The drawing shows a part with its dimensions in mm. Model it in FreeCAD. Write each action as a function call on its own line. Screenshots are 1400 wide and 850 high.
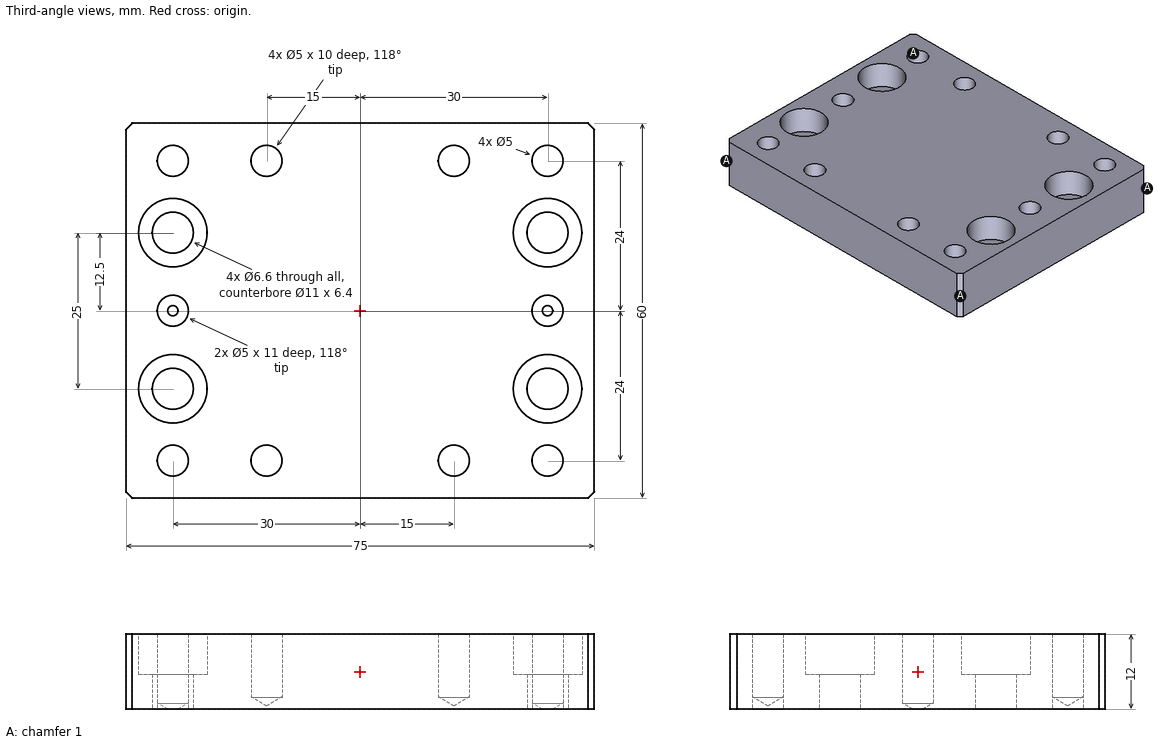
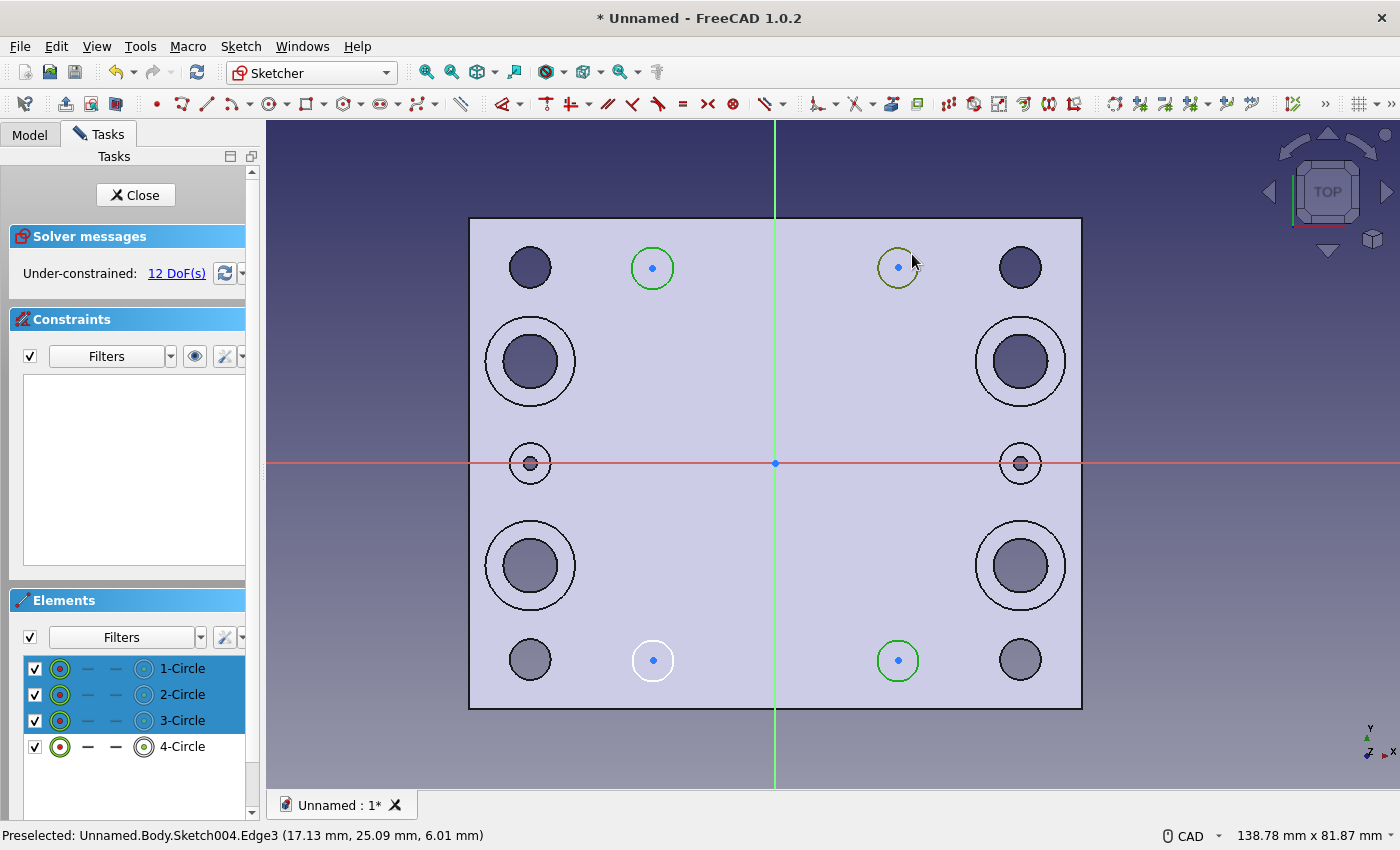
click(667, 646)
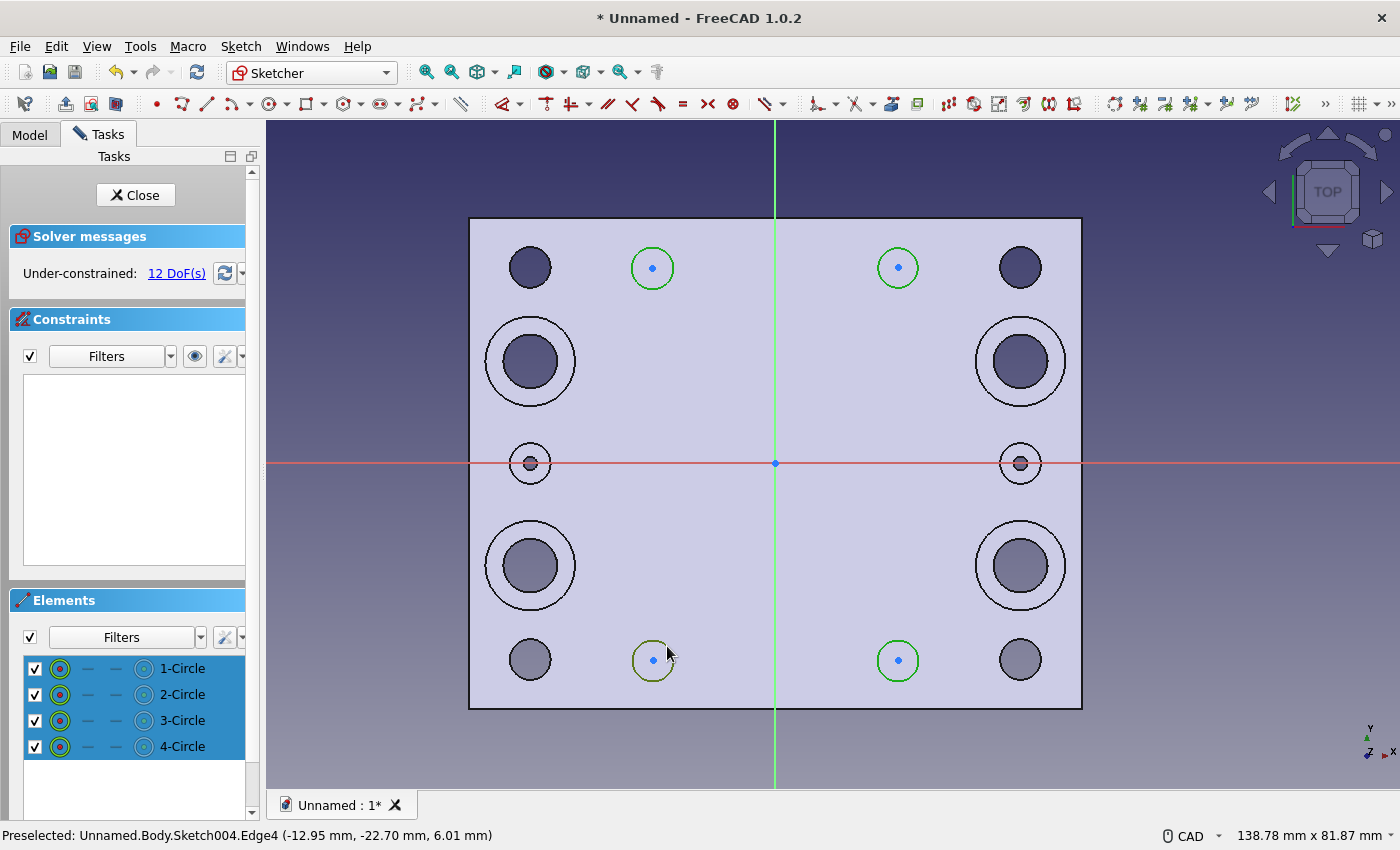
key(e)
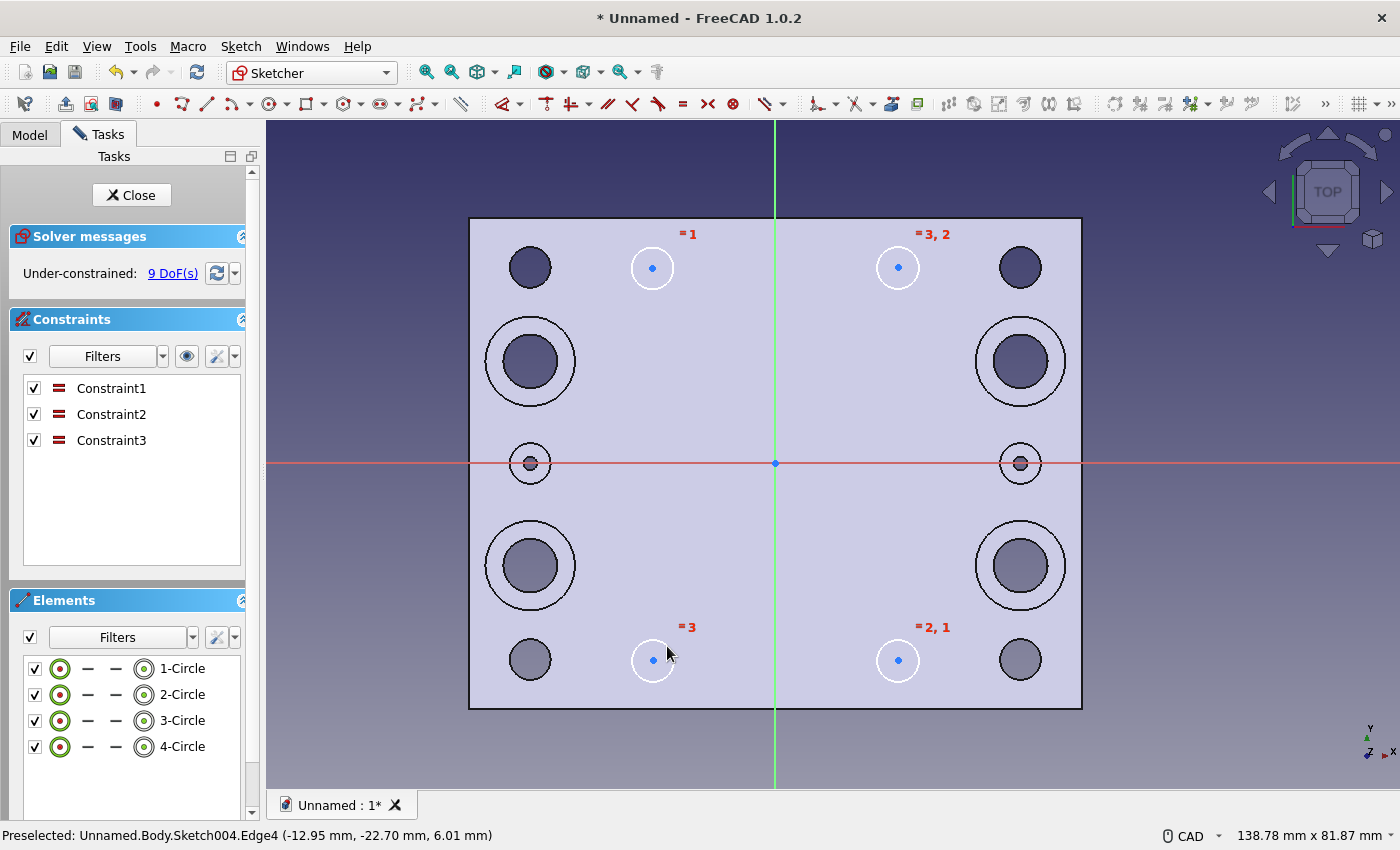
key(d)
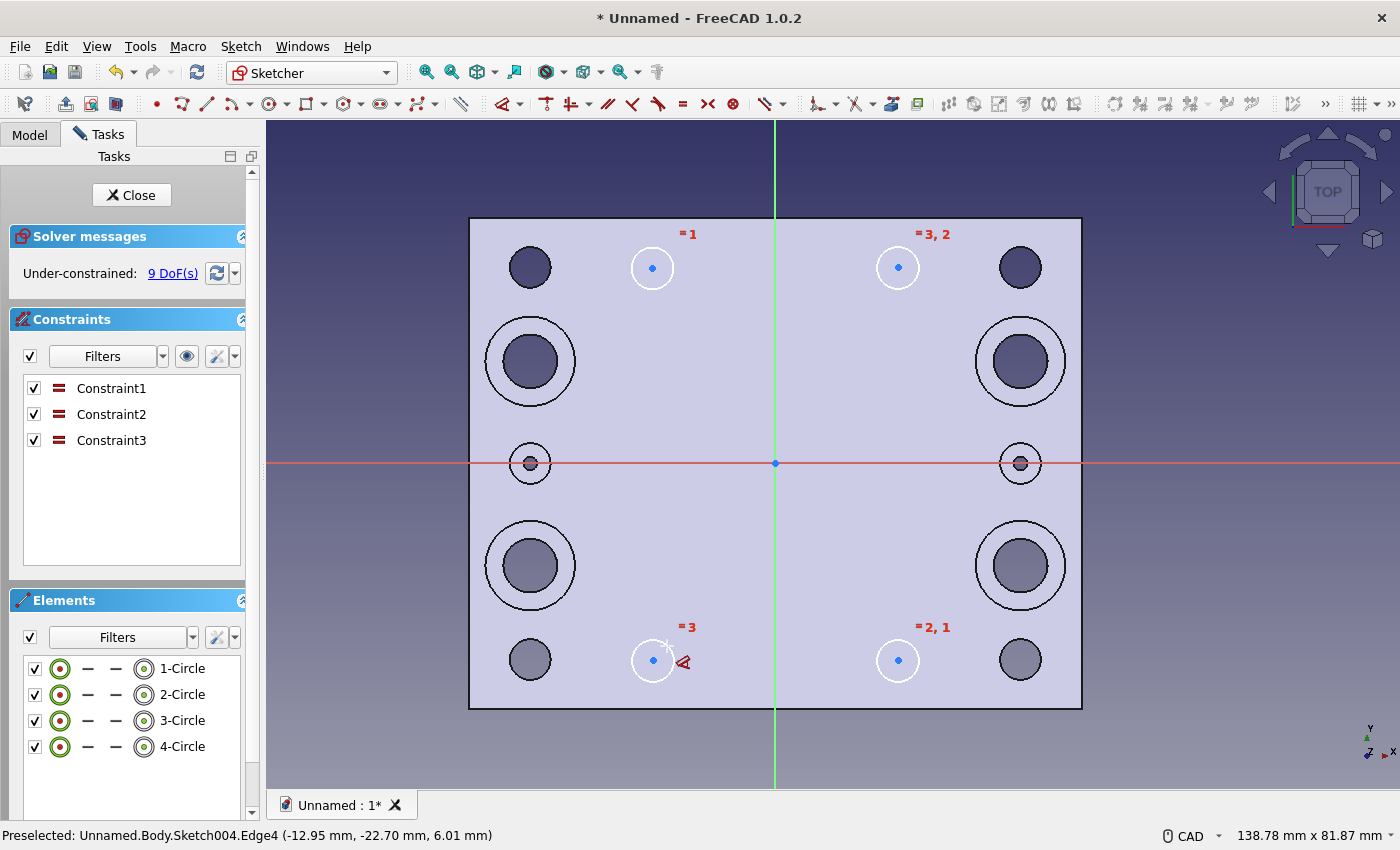
click(667, 254)
click(690, 231)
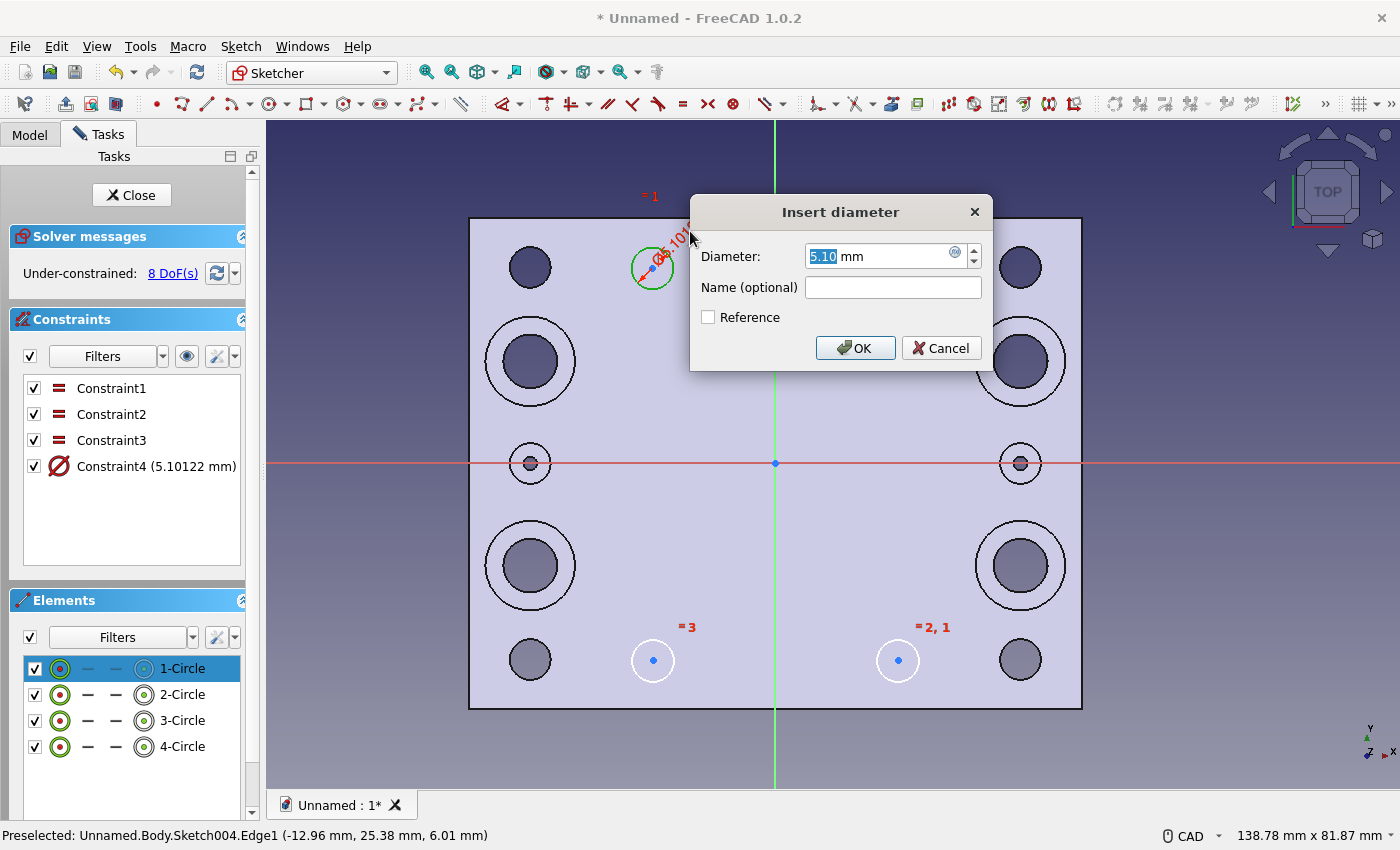
text(5)
key(Return)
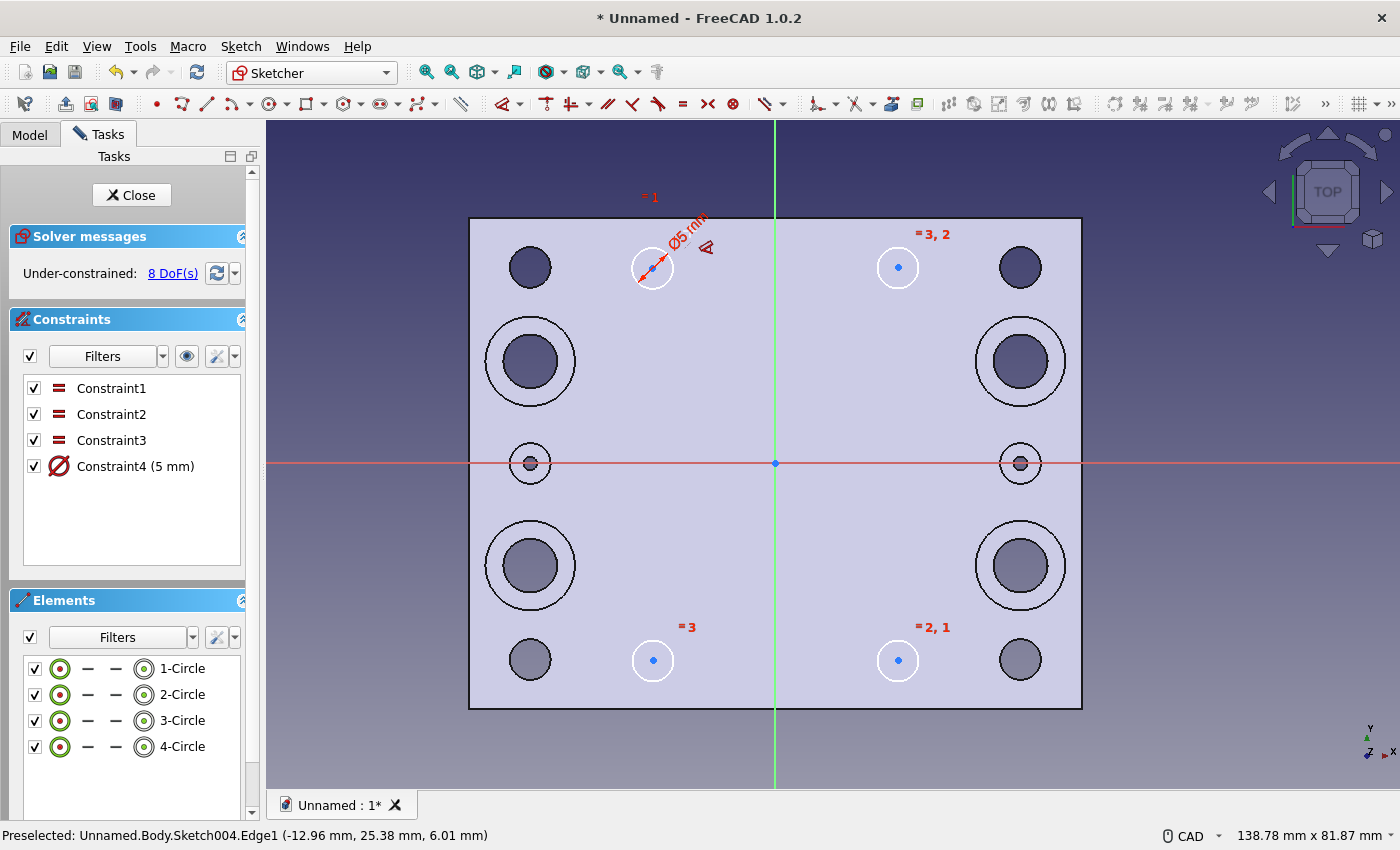
click(653, 268)
click(714, 497)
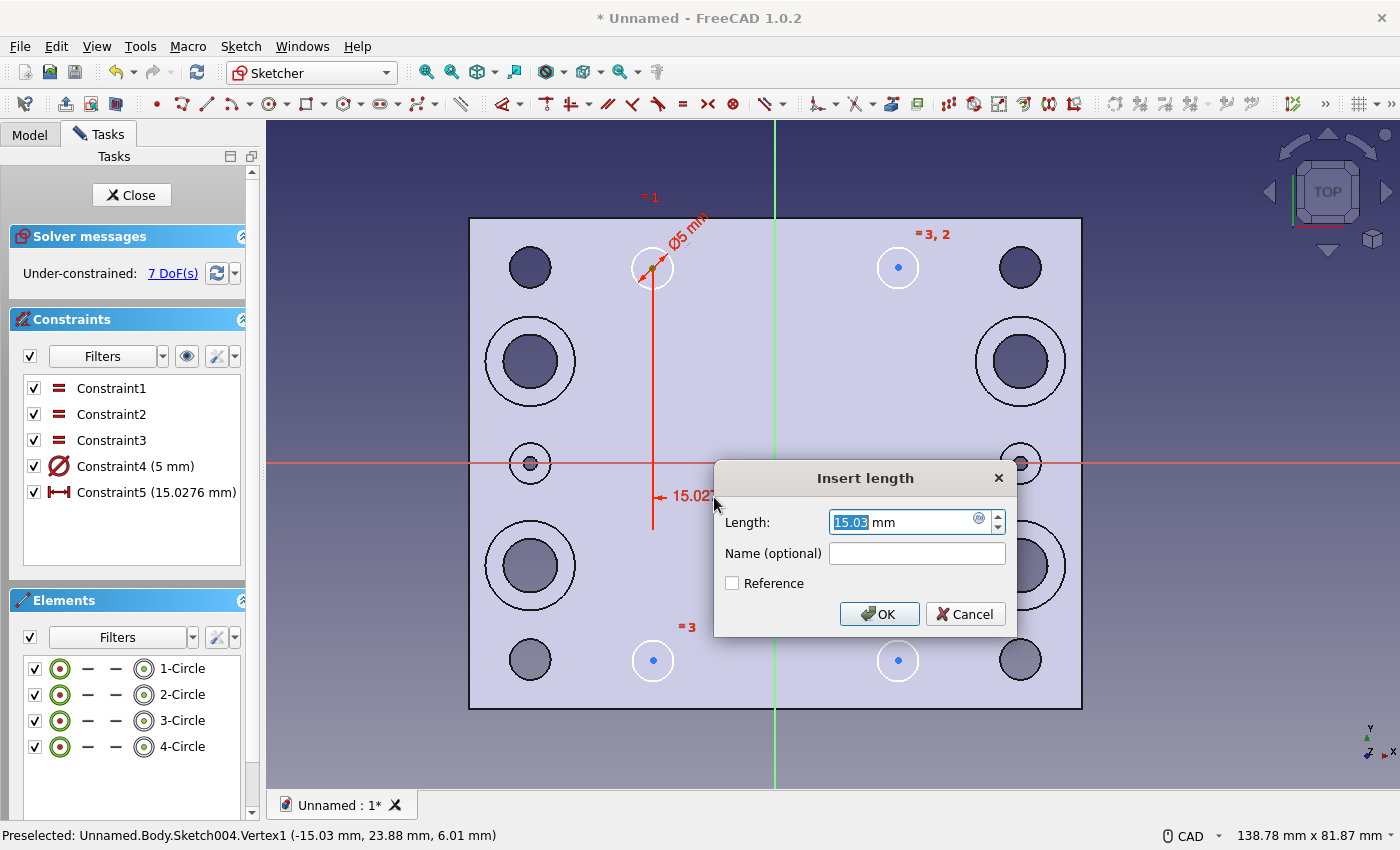
text(15)
key(Return)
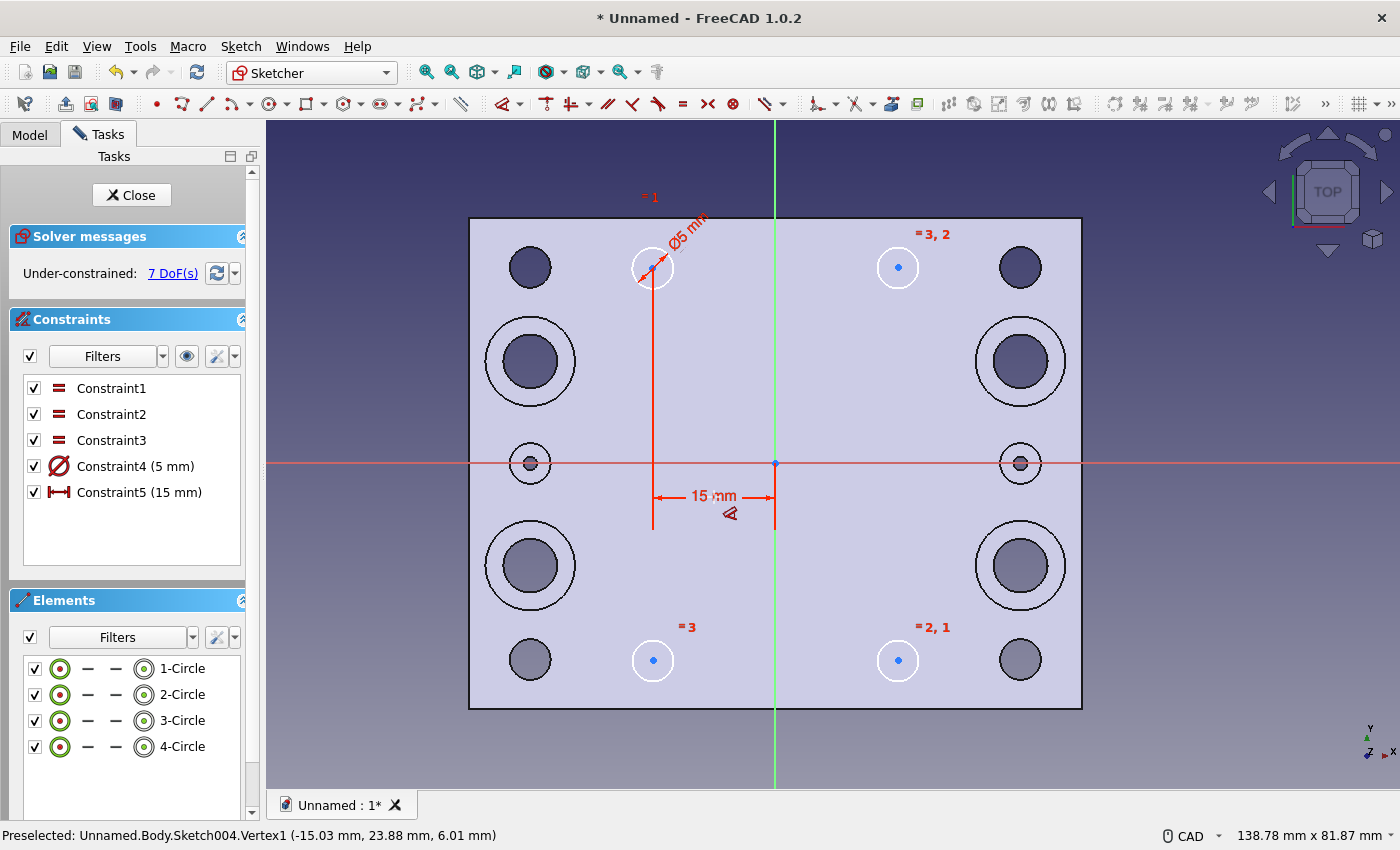
click(653, 268)
click(619, 366)